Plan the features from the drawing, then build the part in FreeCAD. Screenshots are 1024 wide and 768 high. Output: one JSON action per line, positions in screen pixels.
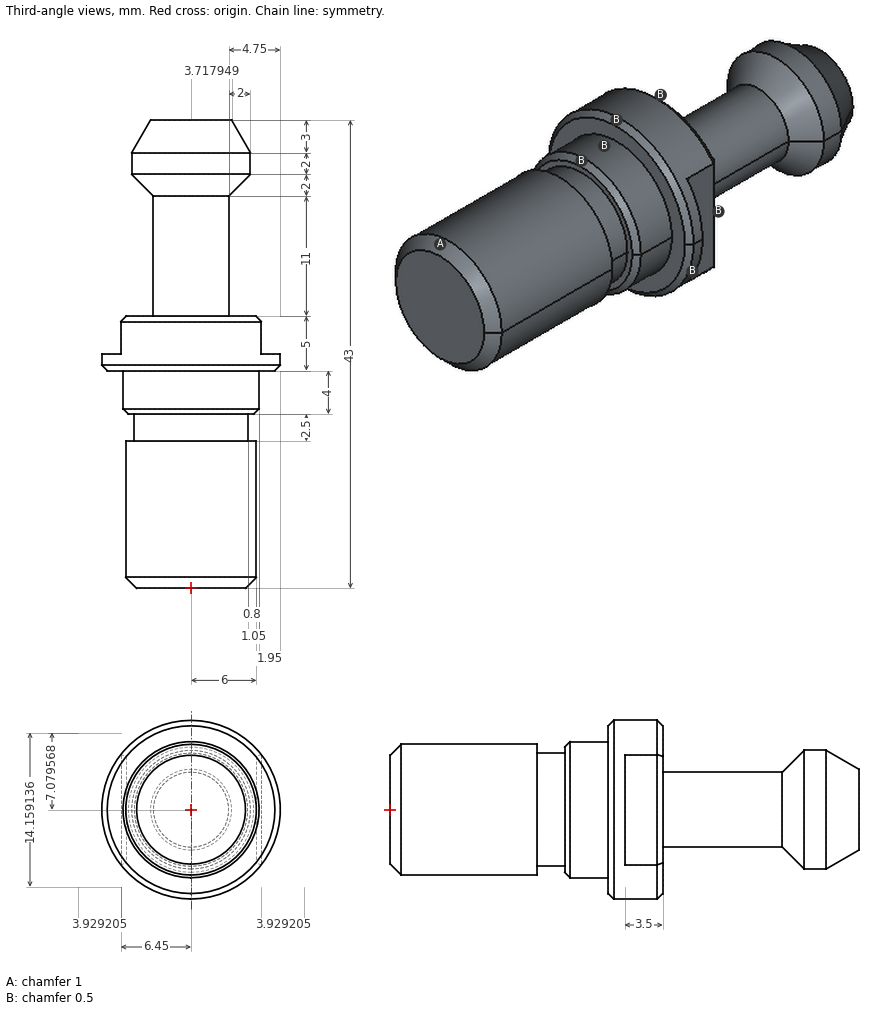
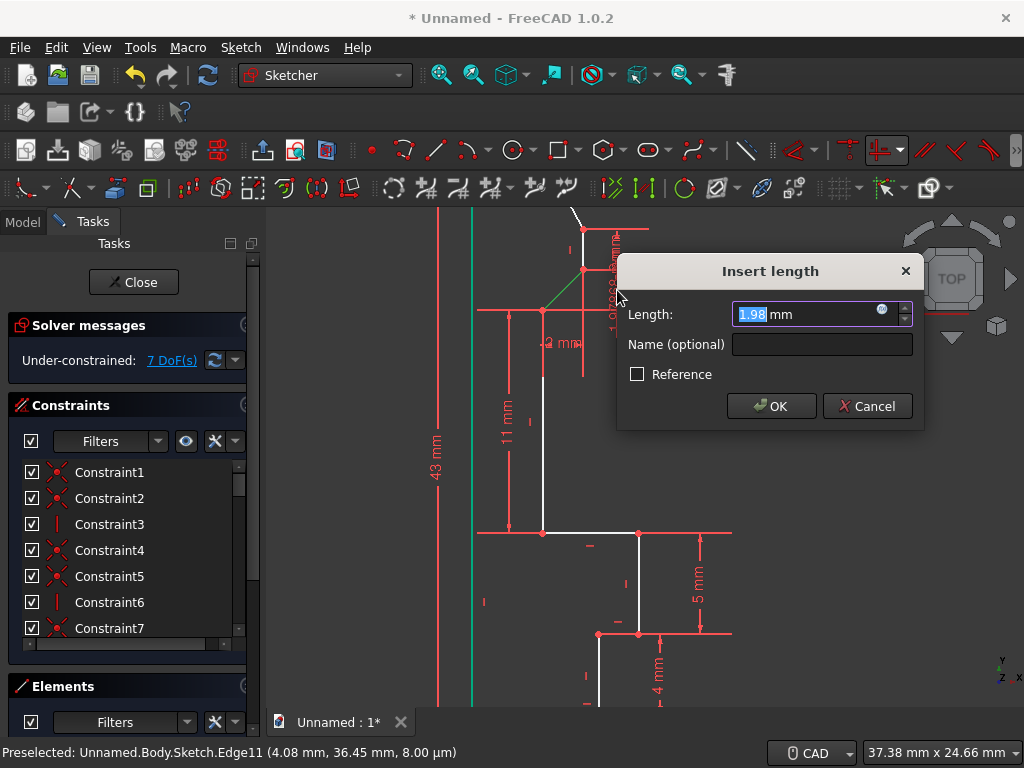
{"action": "type", "text": "2"}
{"action": "key", "text": "Return"}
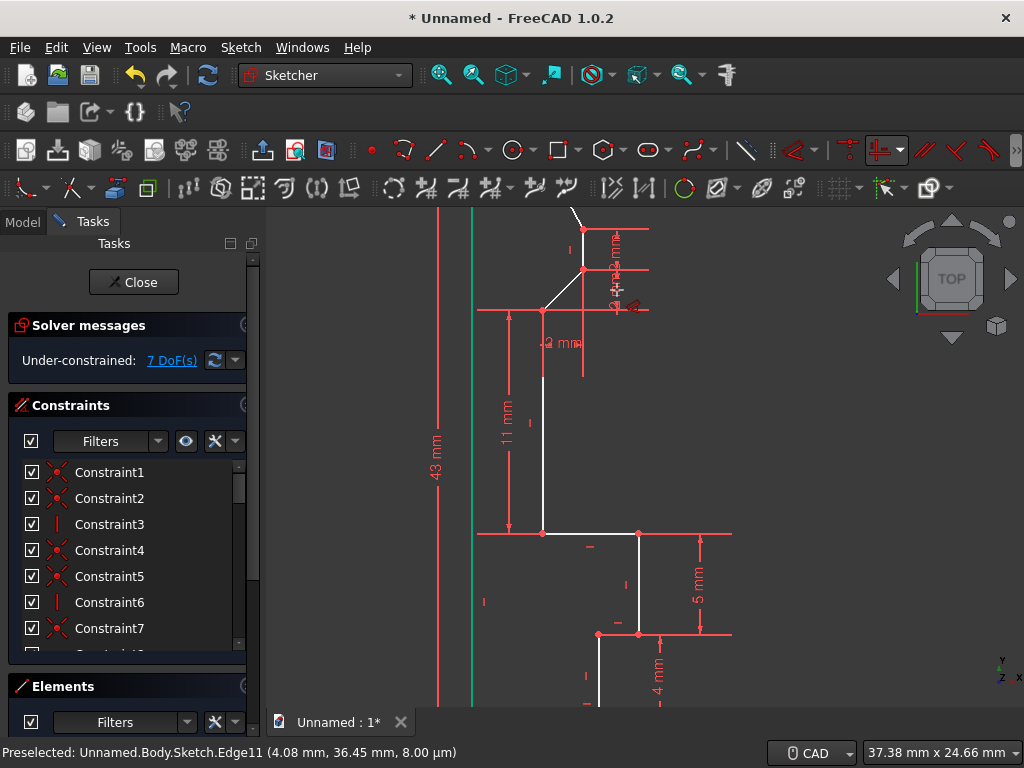
{"action": "scroll", "coordinate": [589, 373], "scroll_direction": "down", "scroll_amount": 5}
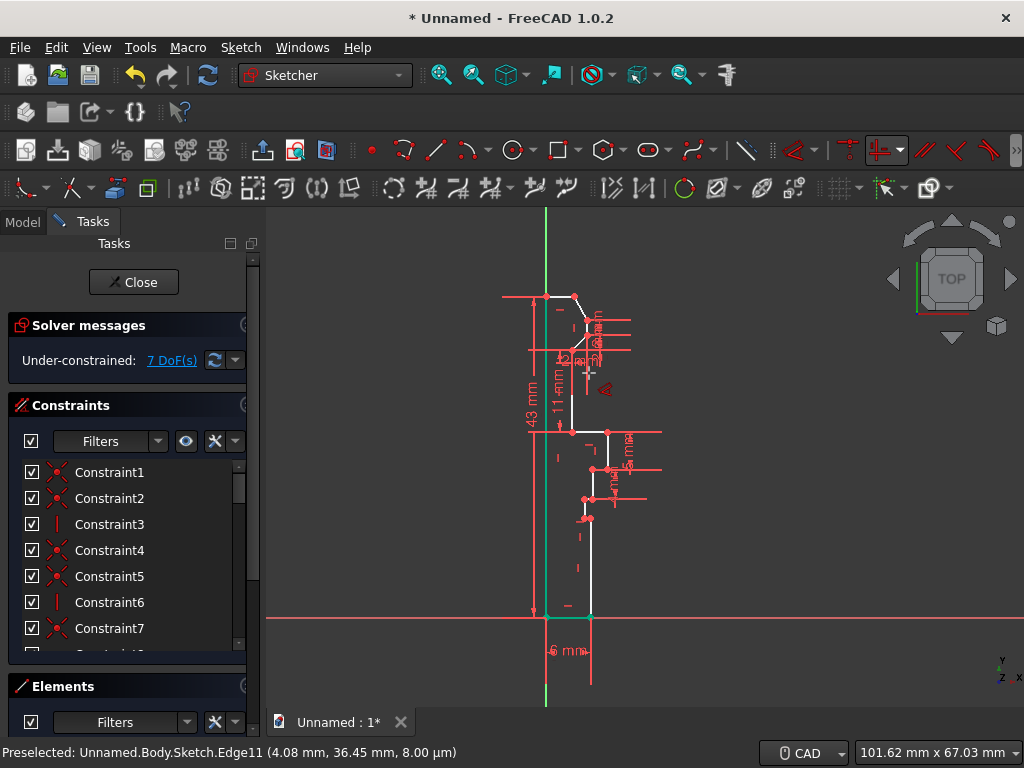
{"action": "scroll", "coordinate": [583, 313], "scroll_direction": "up", "scroll_amount": 3}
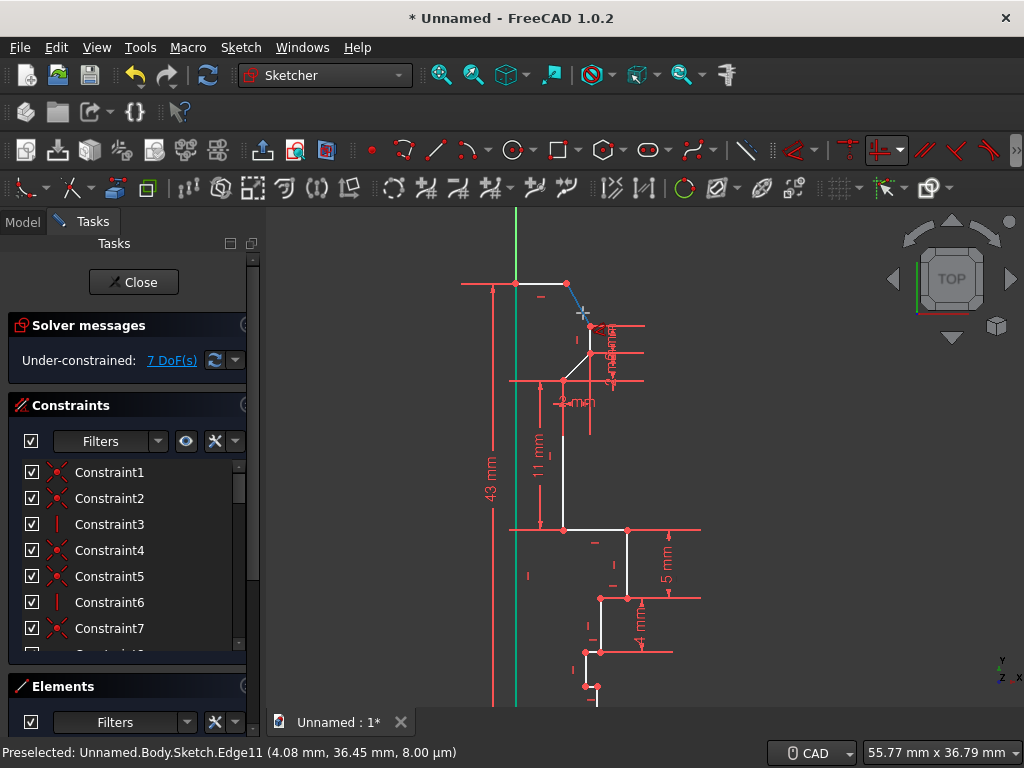
{"action": "left_click", "coordinate": [583, 313]}
{"action": "left_click", "coordinate": [624, 305]}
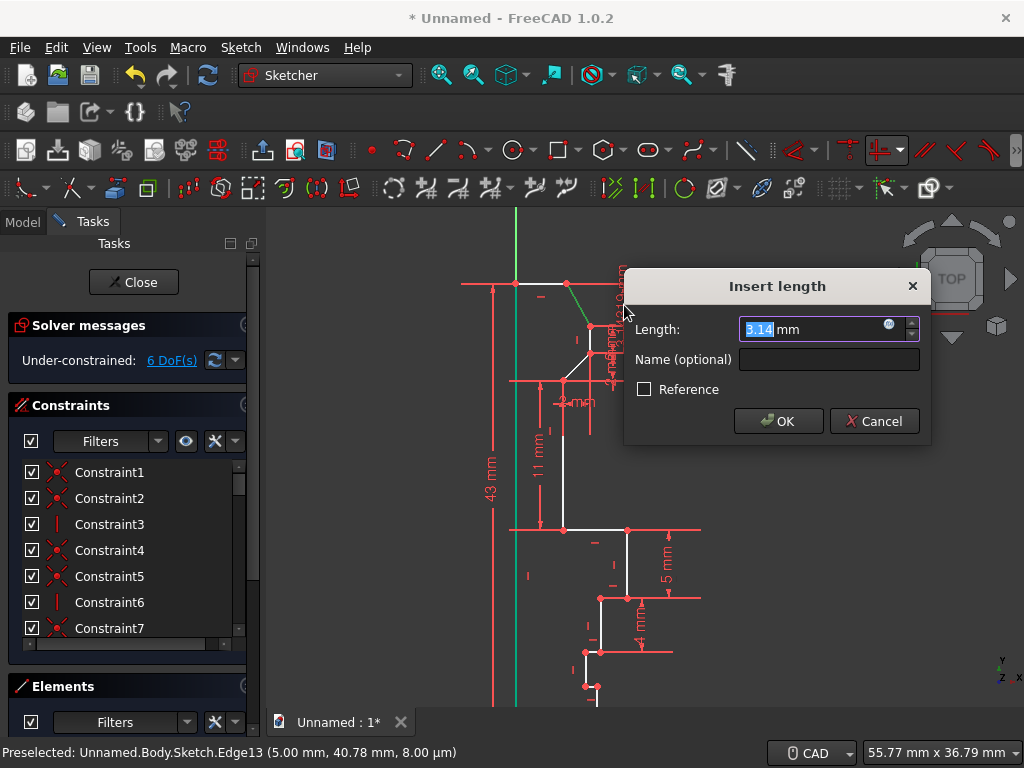
{"action": "type", "text": "3"}
{"action": "key", "text": "Return"}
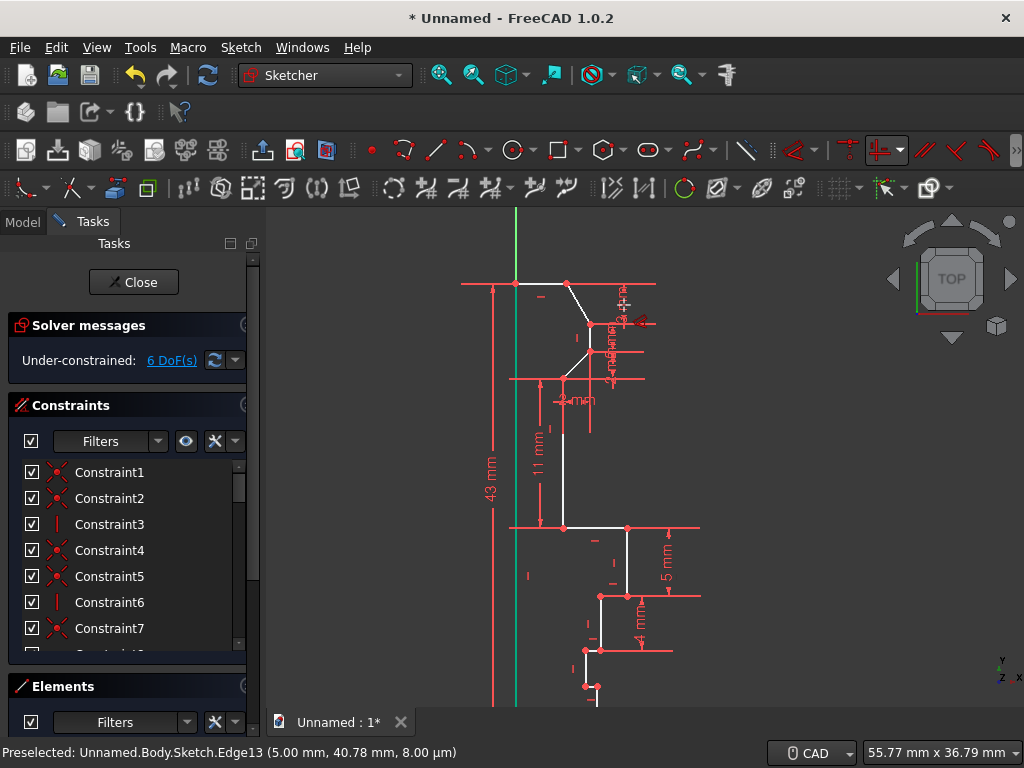
{"action": "scroll", "coordinate": [583, 313], "scroll_direction": "down", "scroll_amount": 3}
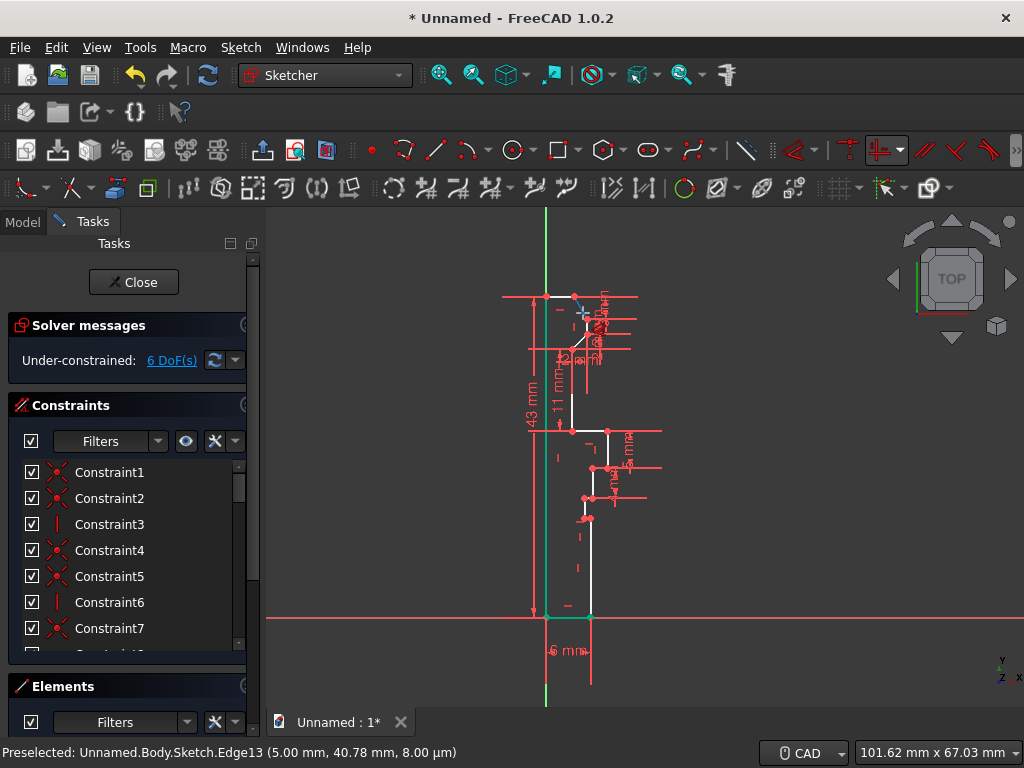
{"action": "scroll", "coordinate": [588, 518], "scroll_direction": "up", "scroll_amount": 10}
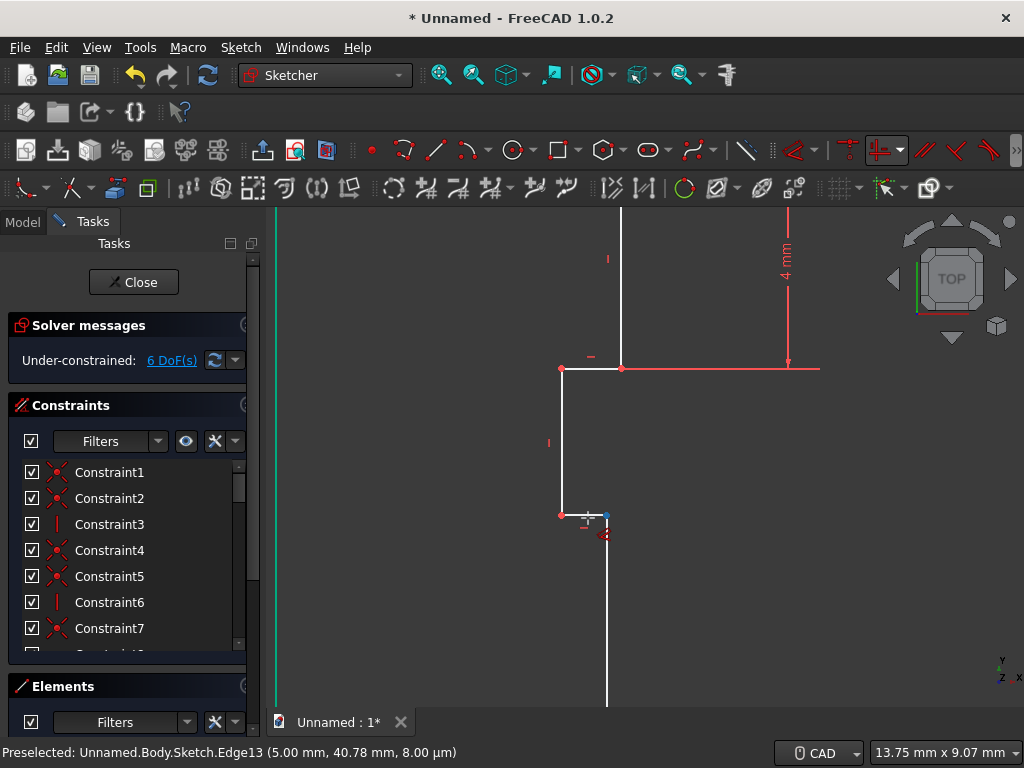
{"action": "left_click", "coordinate": [584, 515]}
{"action": "left_click", "coordinate": [584, 549]}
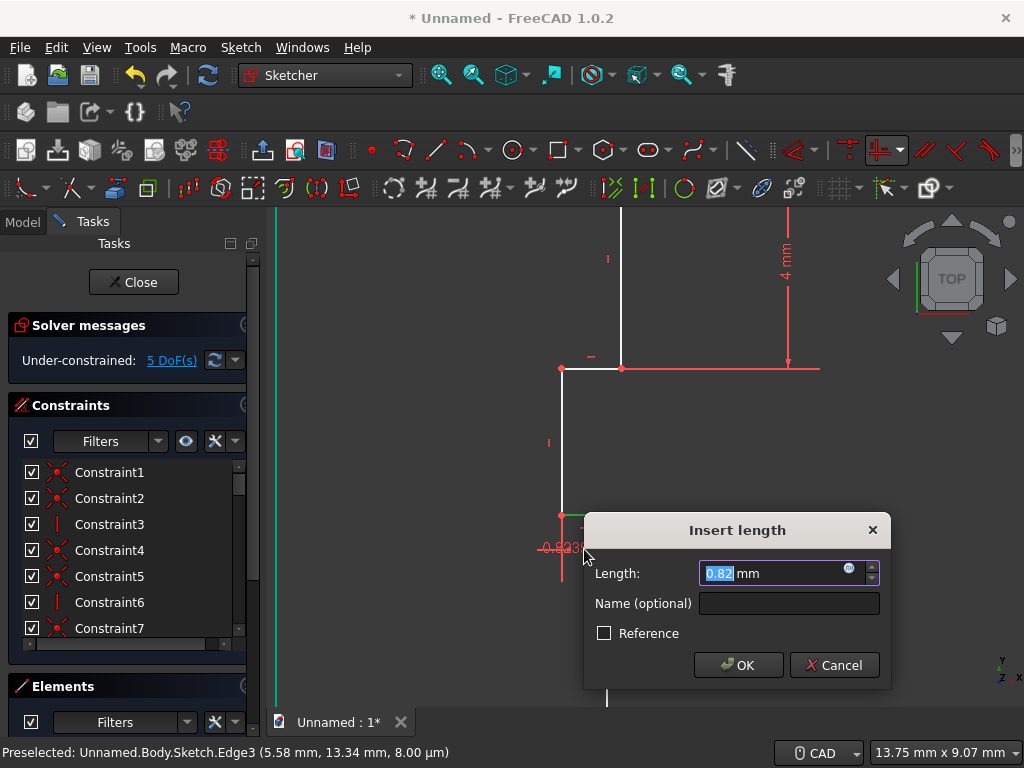
{"action": "type", "text": "0.8"}
{"action": "key", "text": "Return"}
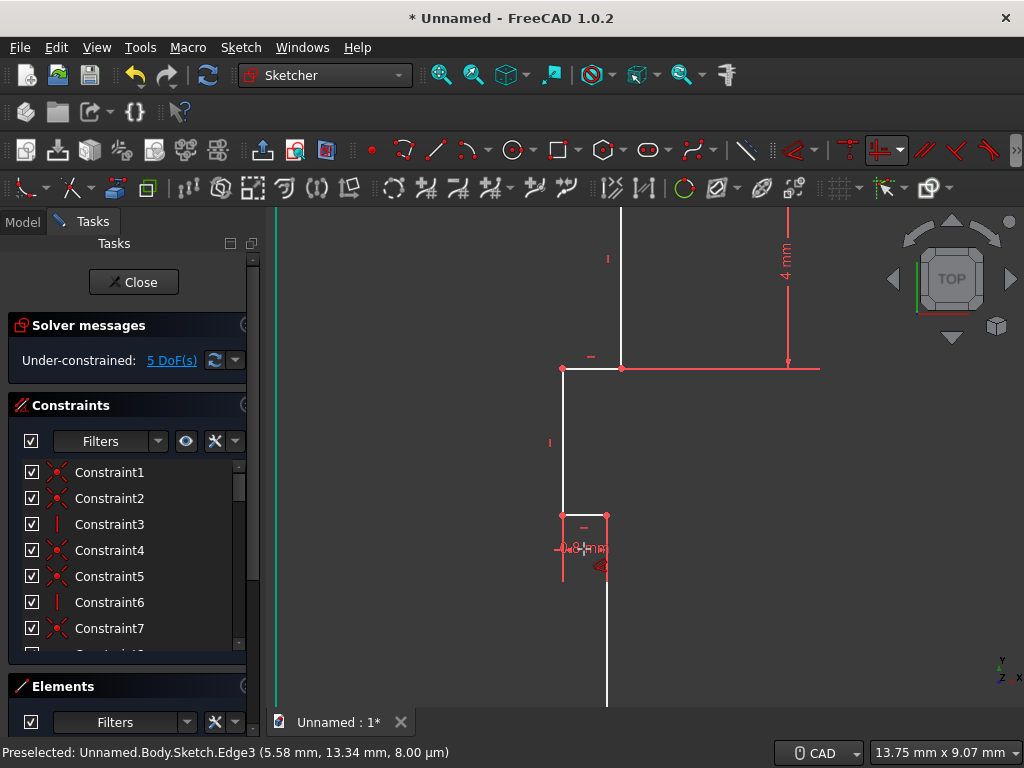
{"action": "scroll", "coordinate": [588, 518], "scroll_direction": "down", "scroll_amount": 10}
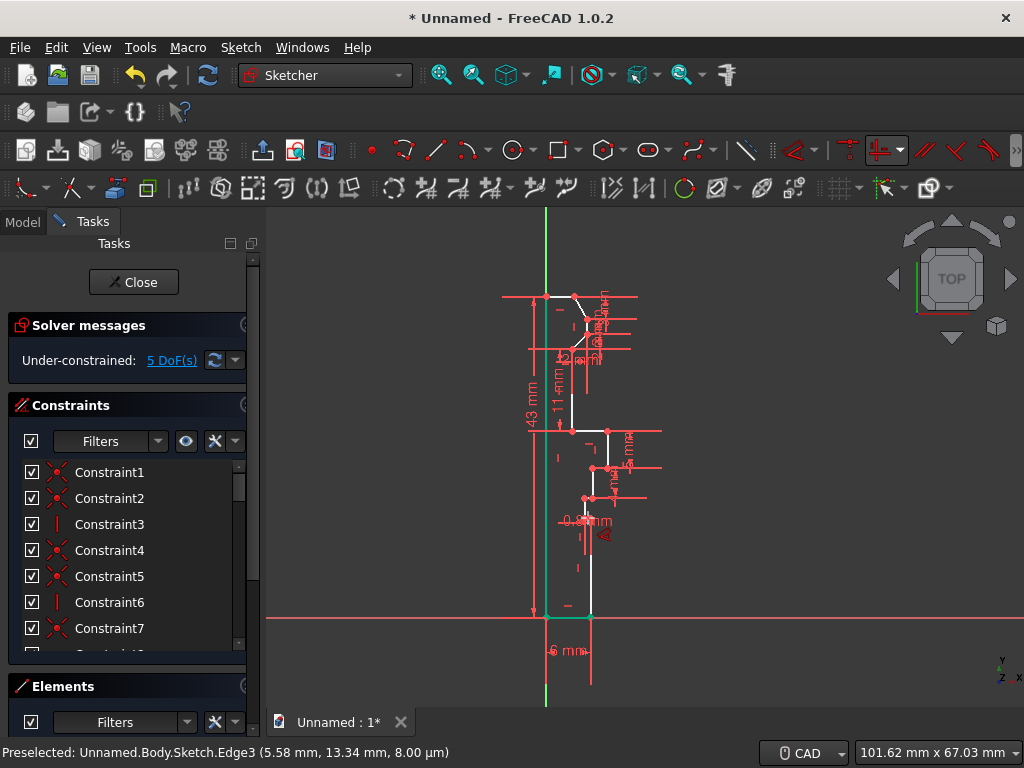
{"action": "scroll", "coordinate": [585, 512], "scroll_direction": "up", "scroll_amount": 5}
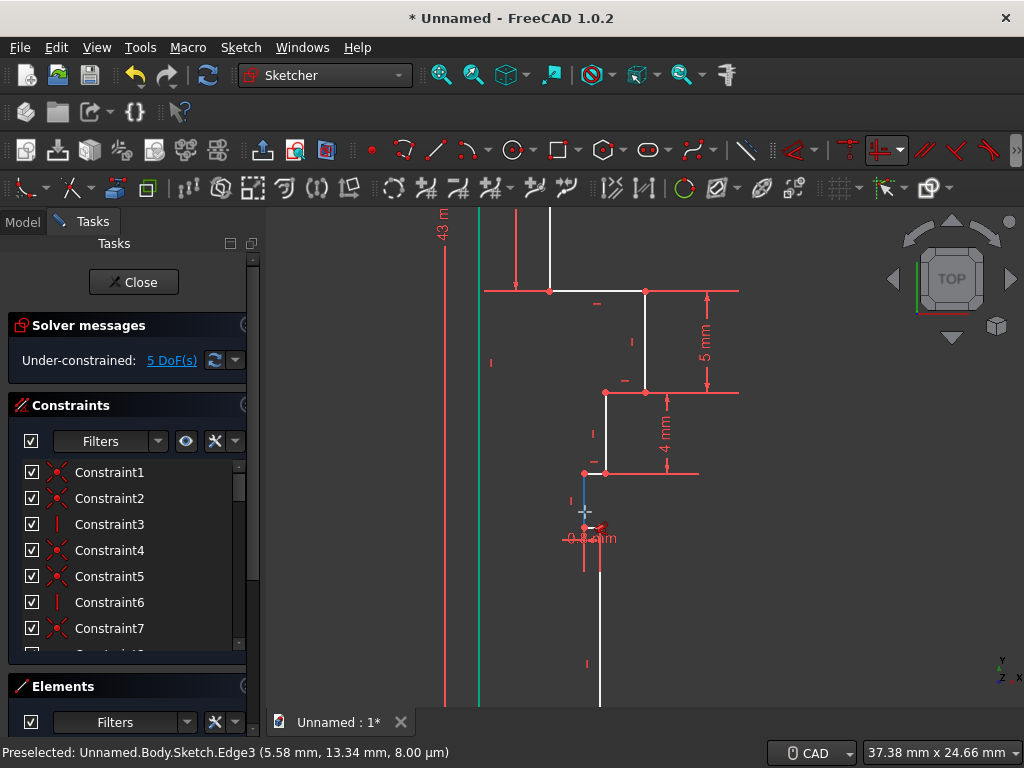
{"action": "left_click", "coordinate": [584, 512]}
{"action": "left_click", "coordinate": [618, 501]}